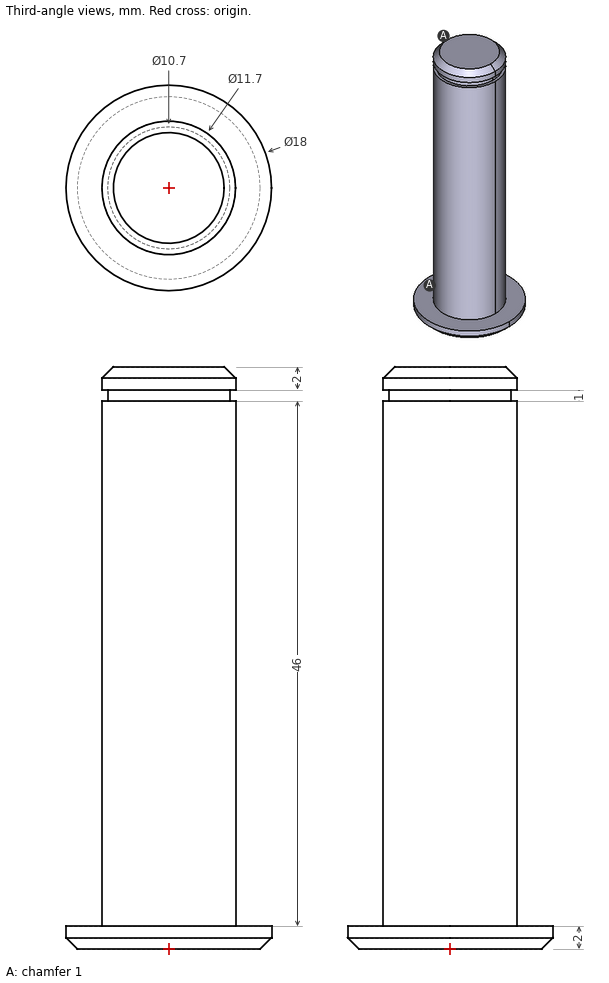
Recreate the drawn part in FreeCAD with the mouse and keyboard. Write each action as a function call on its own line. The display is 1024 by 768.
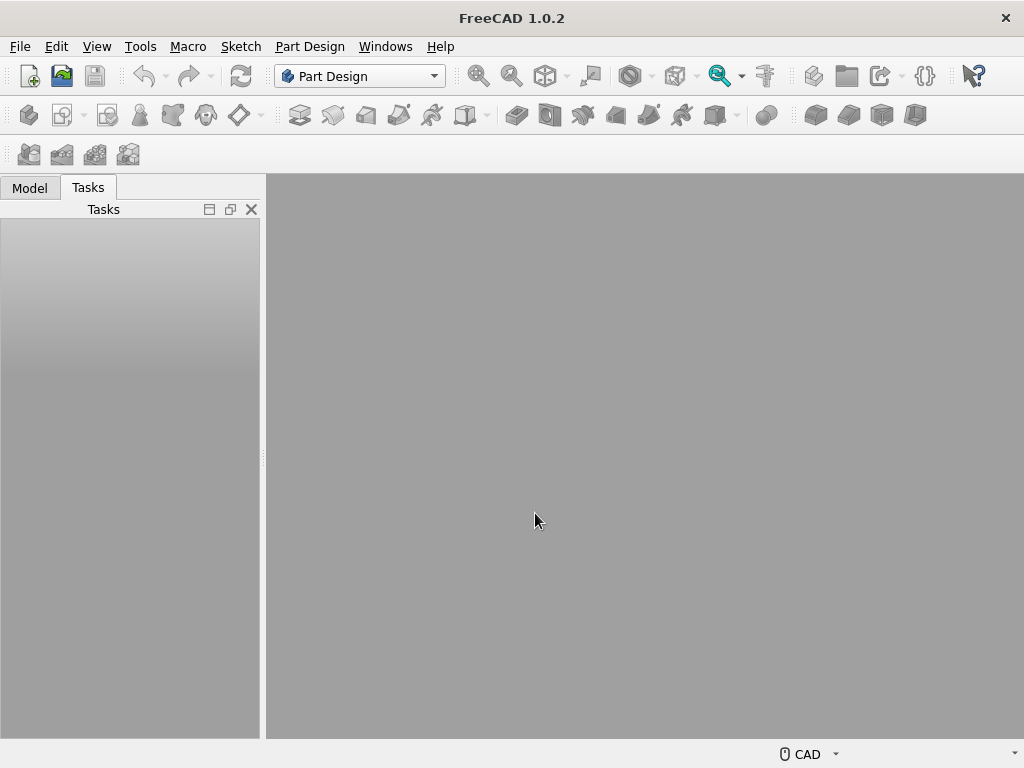
click(29, 76)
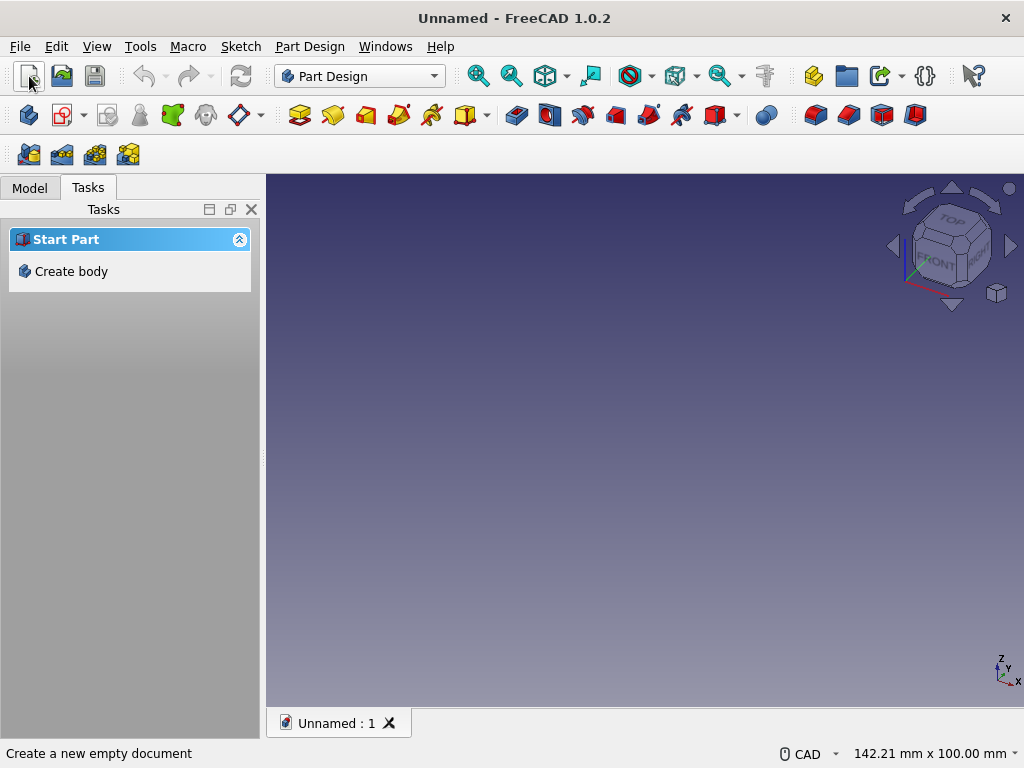
click(62, 116)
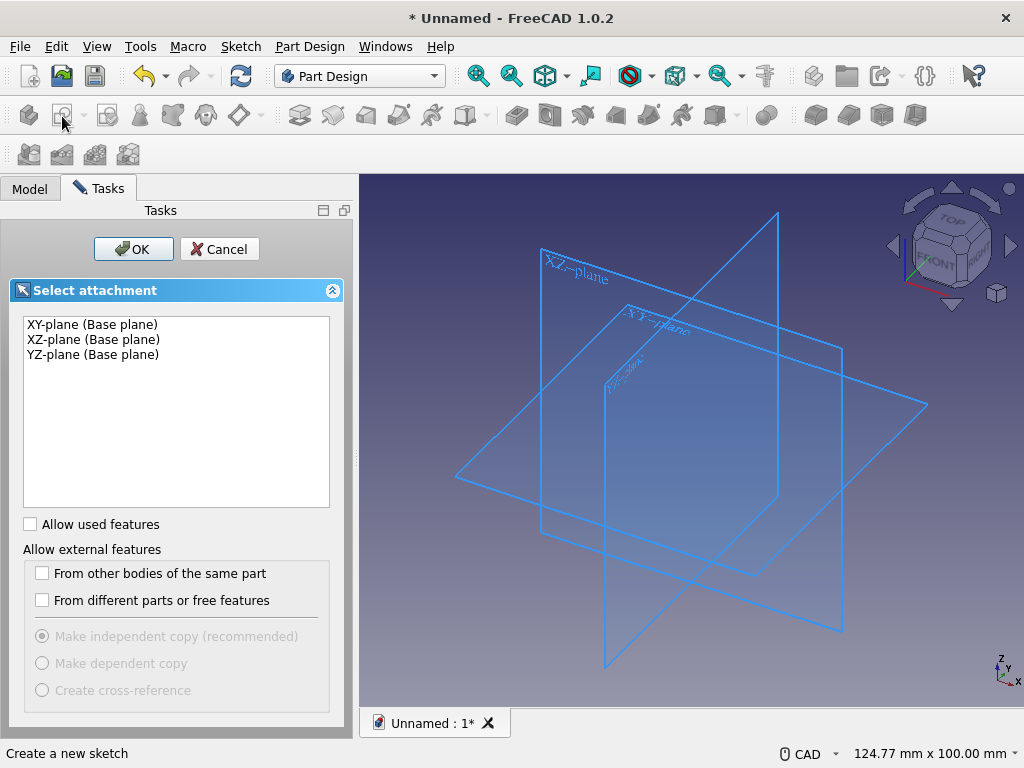
click(84, 324)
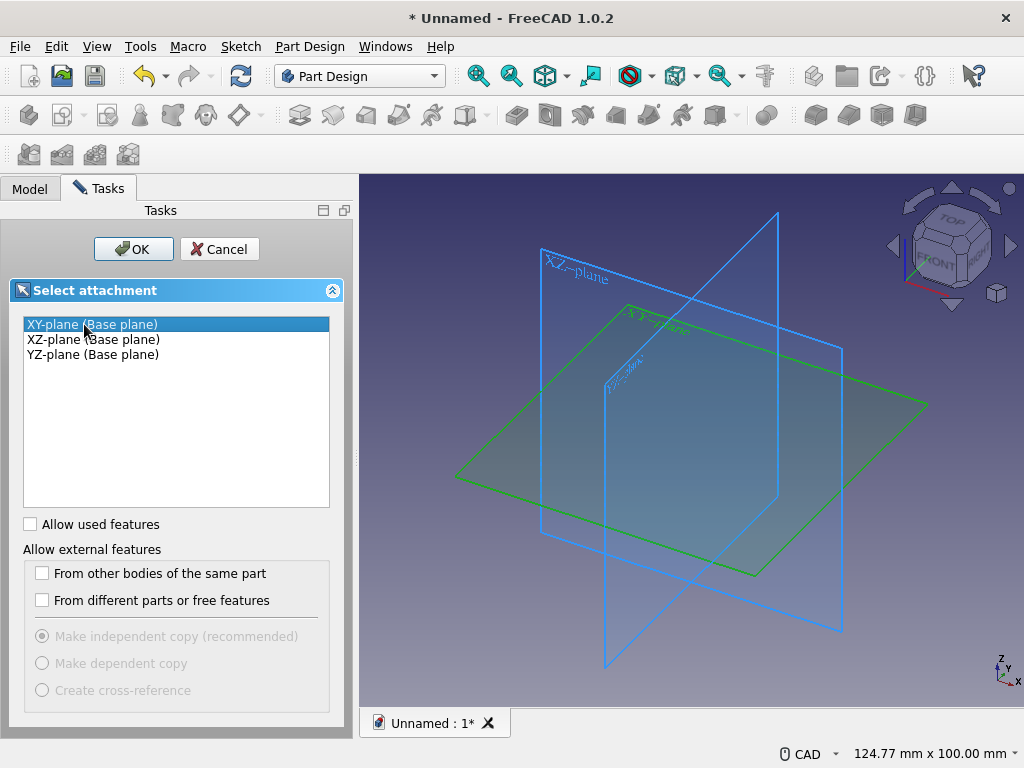
click(134, 249)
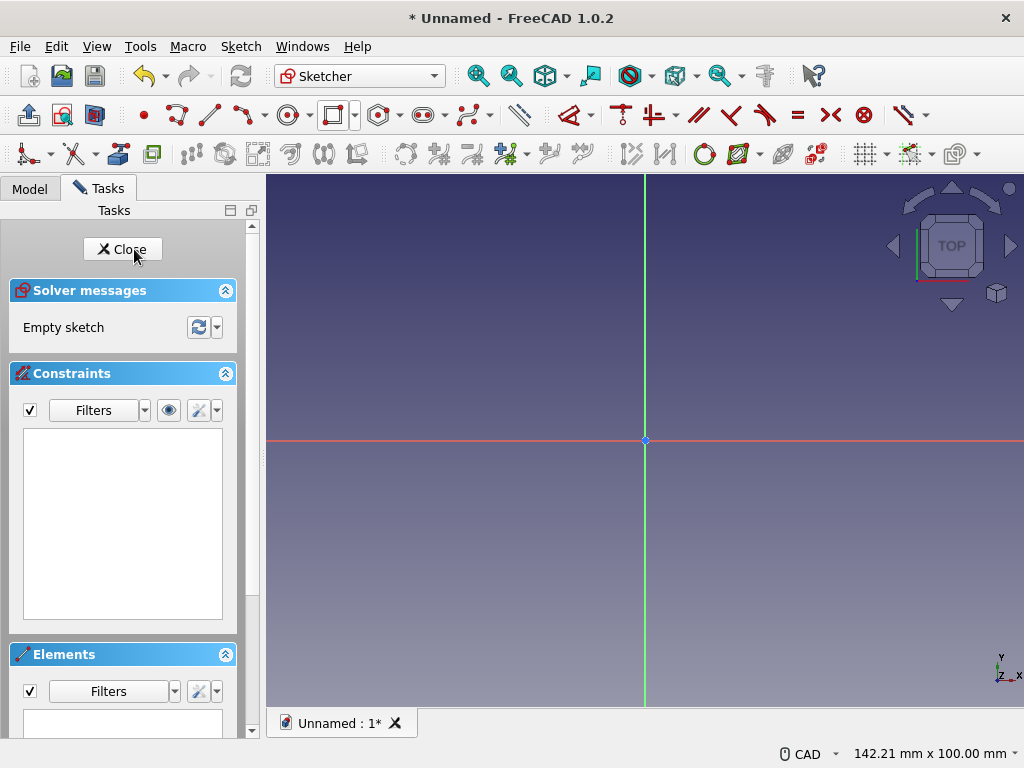
scroll(675, 440, up, 6)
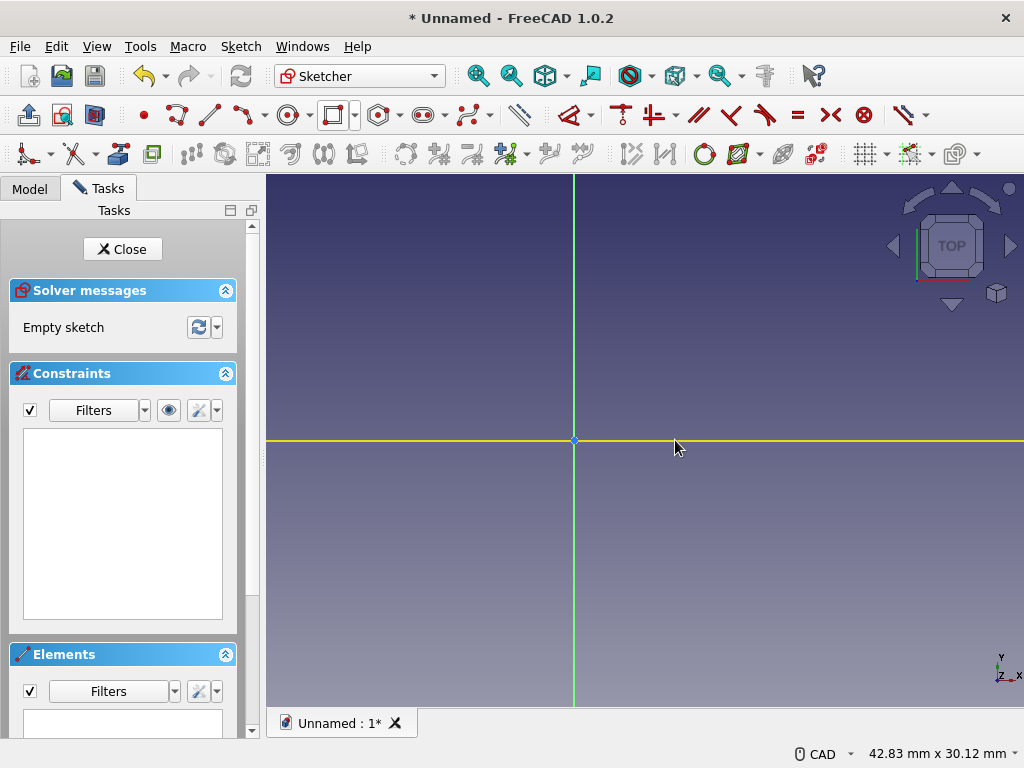
click(288, 116)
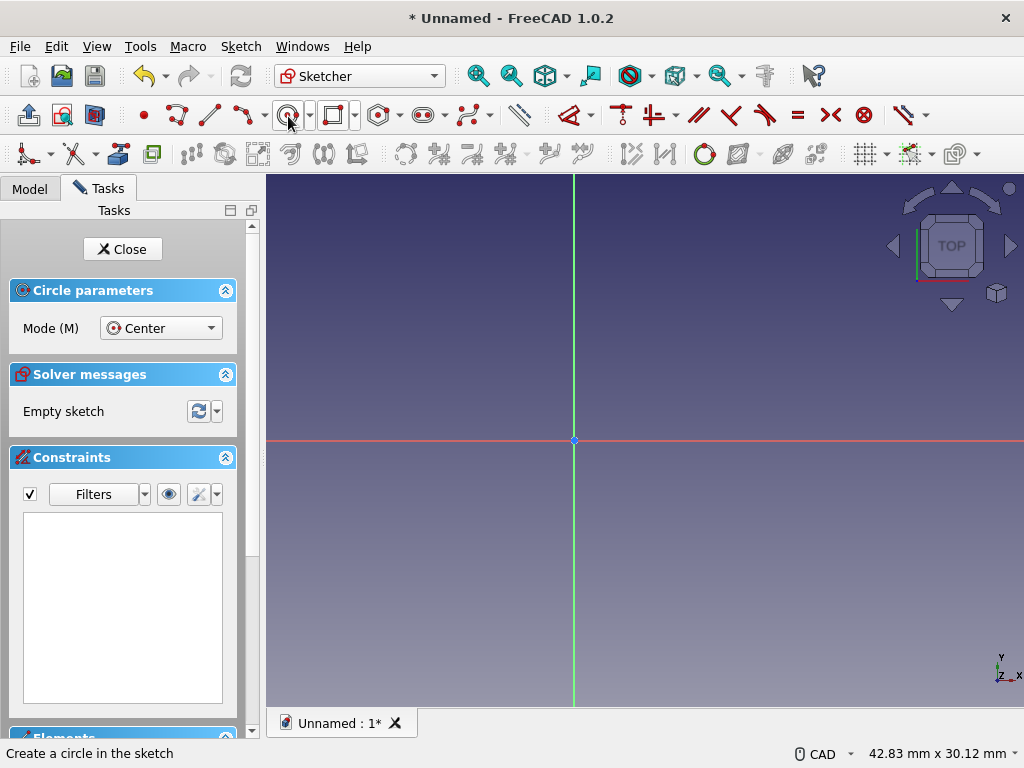
click(574, 440)
move(687, 328)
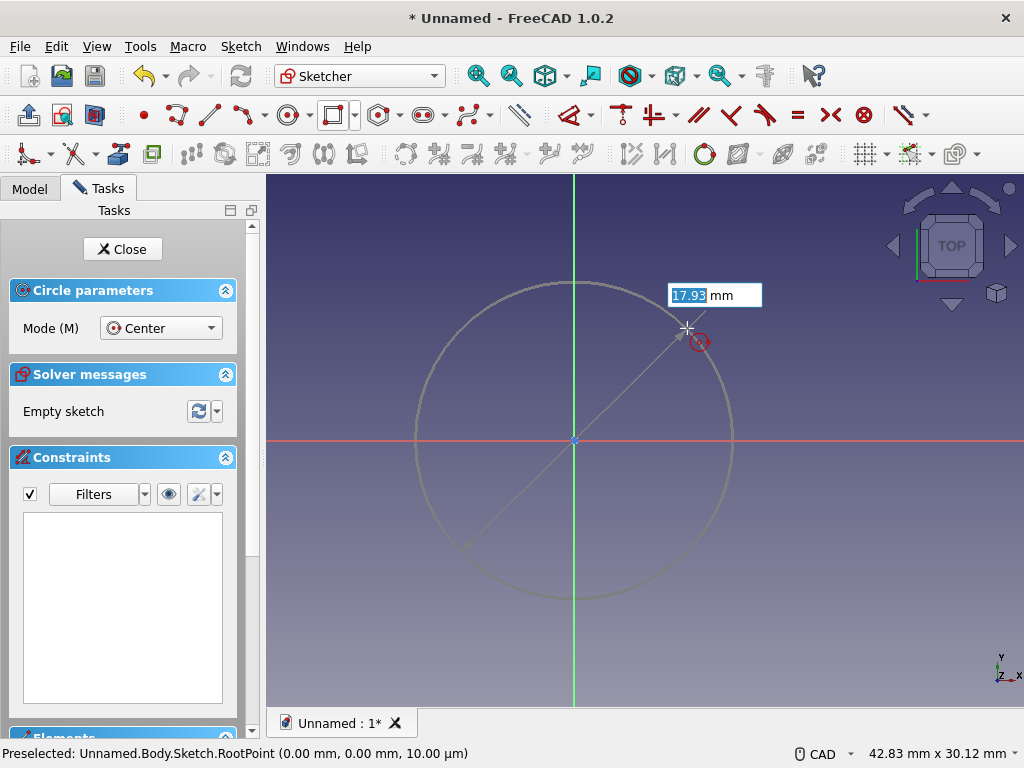
text(18)
key(Return)
key(Escape)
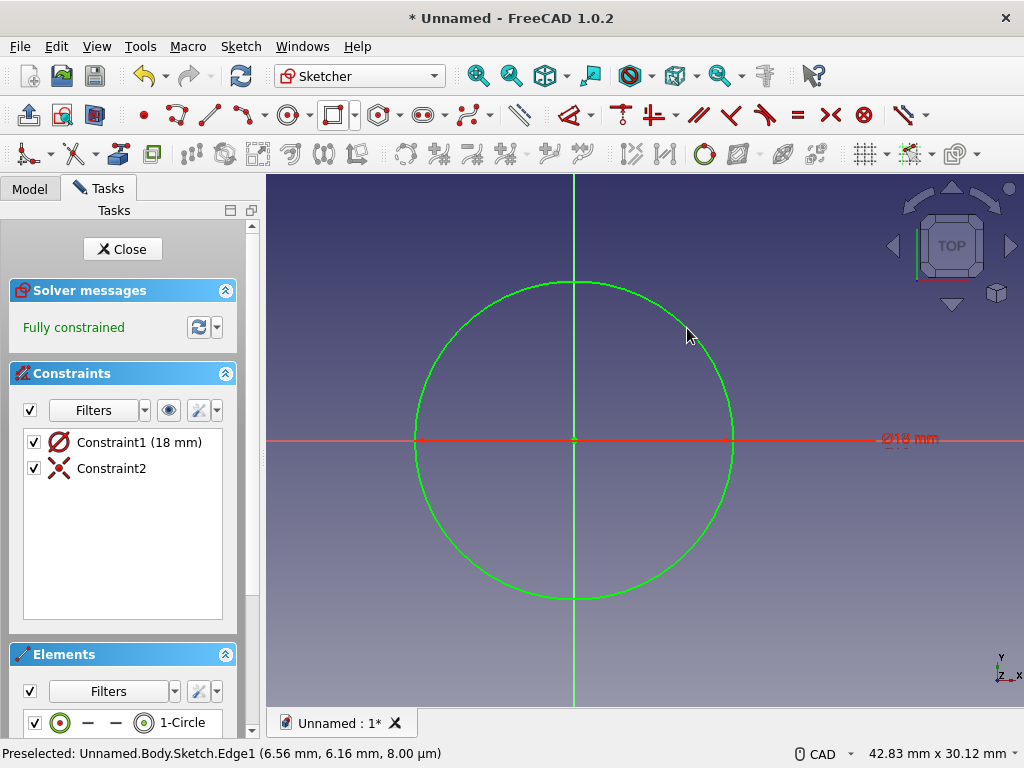
click(123, 249)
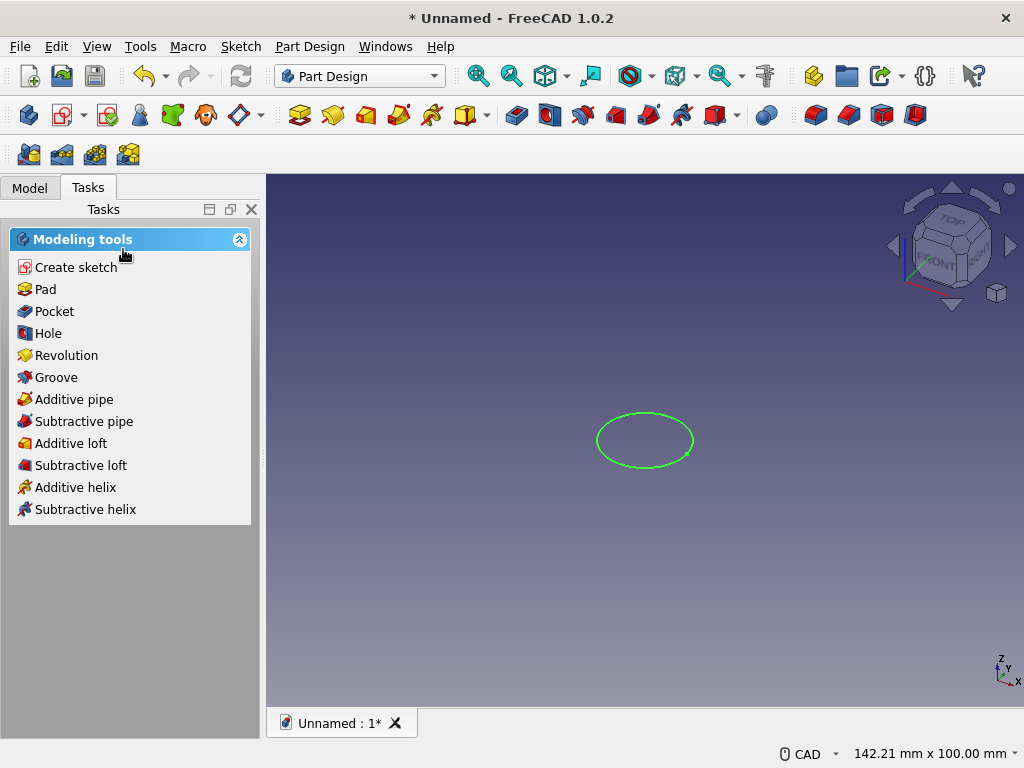
click(300, 116)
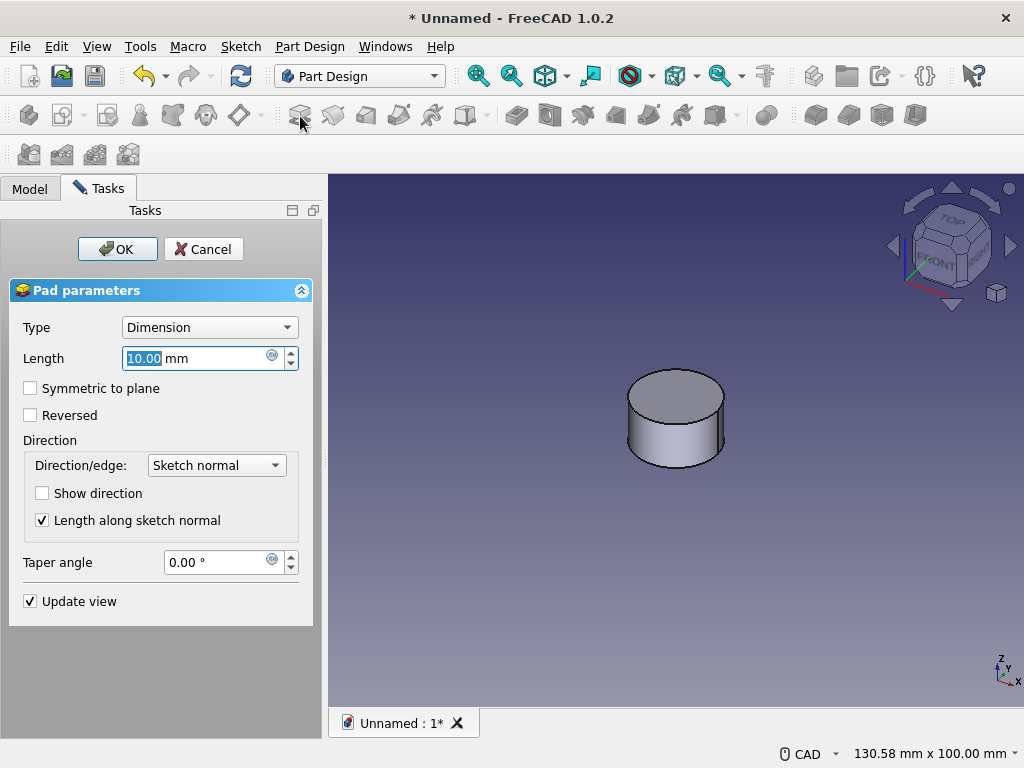
text(2)
key(Tab)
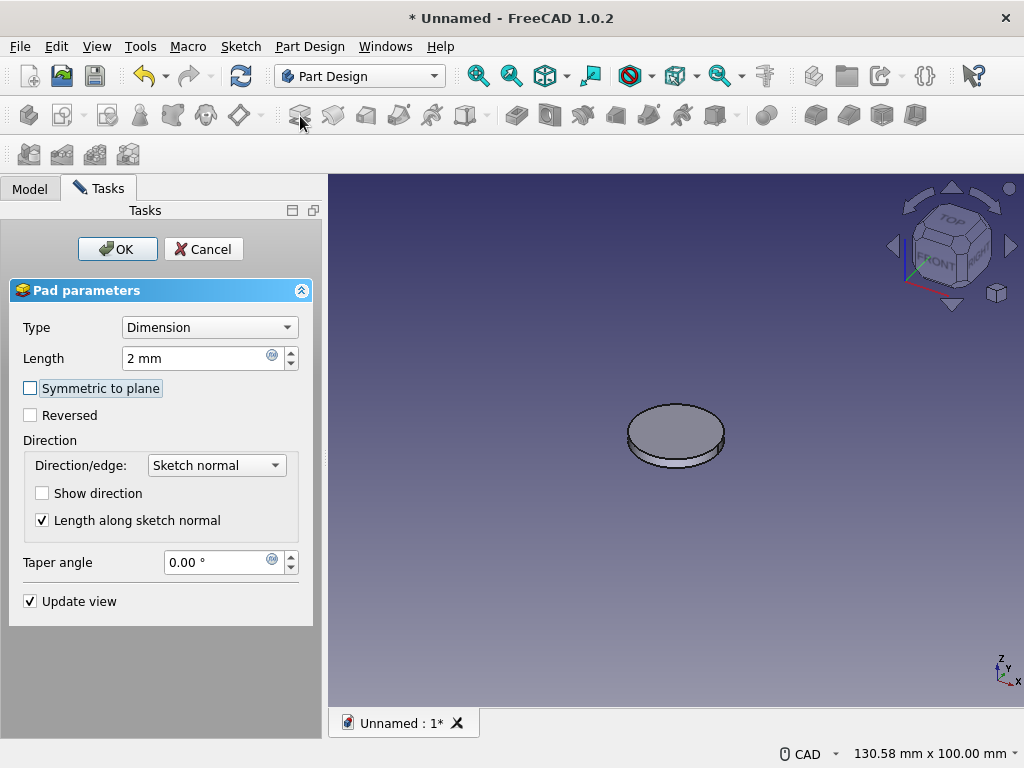
click(118, 249)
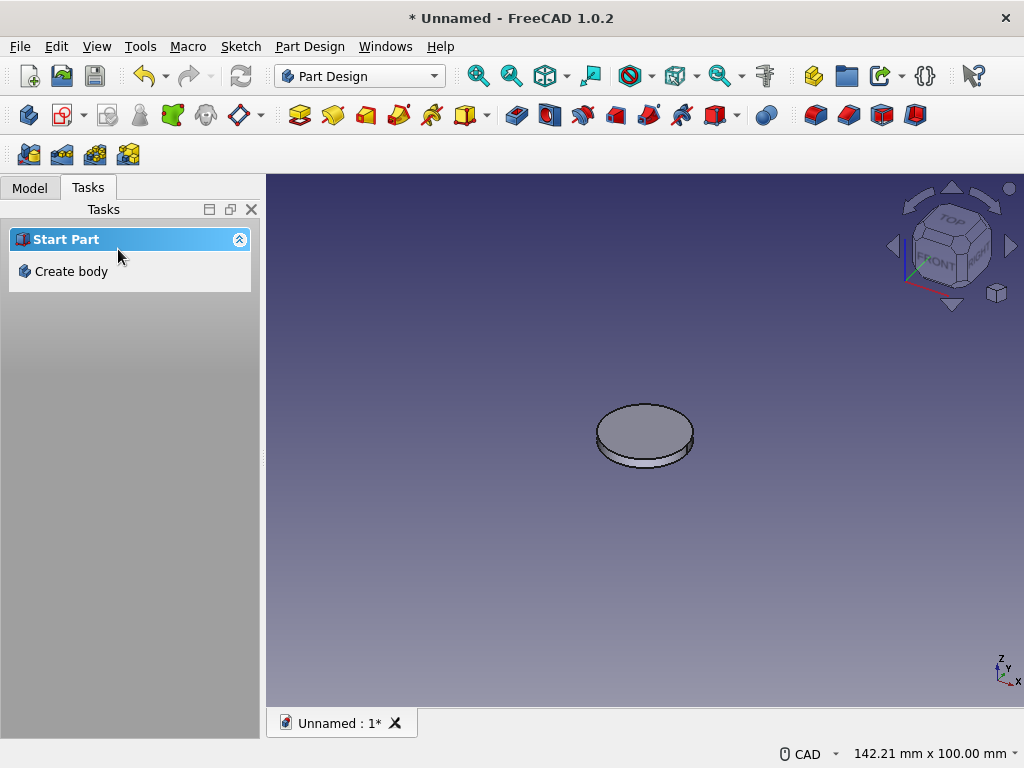
click(479, 76)